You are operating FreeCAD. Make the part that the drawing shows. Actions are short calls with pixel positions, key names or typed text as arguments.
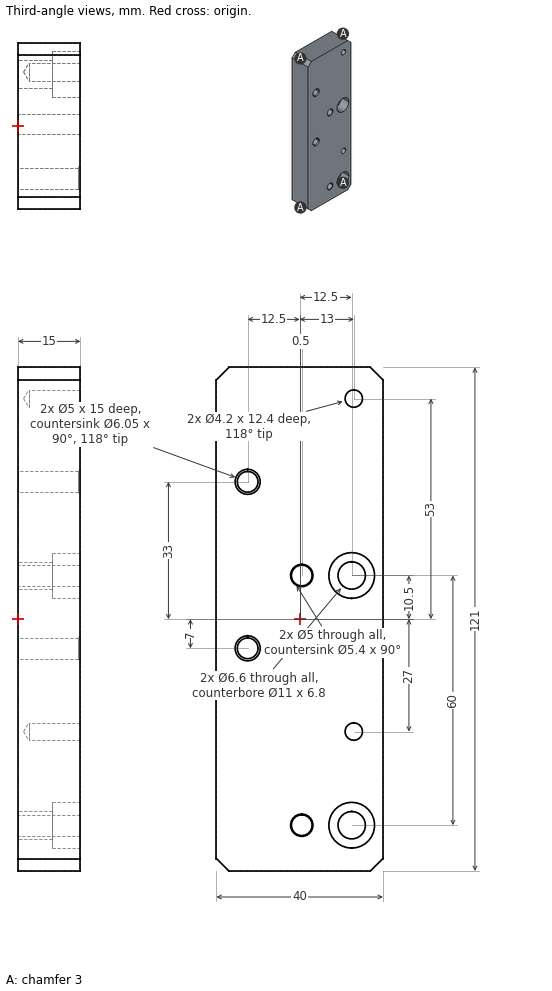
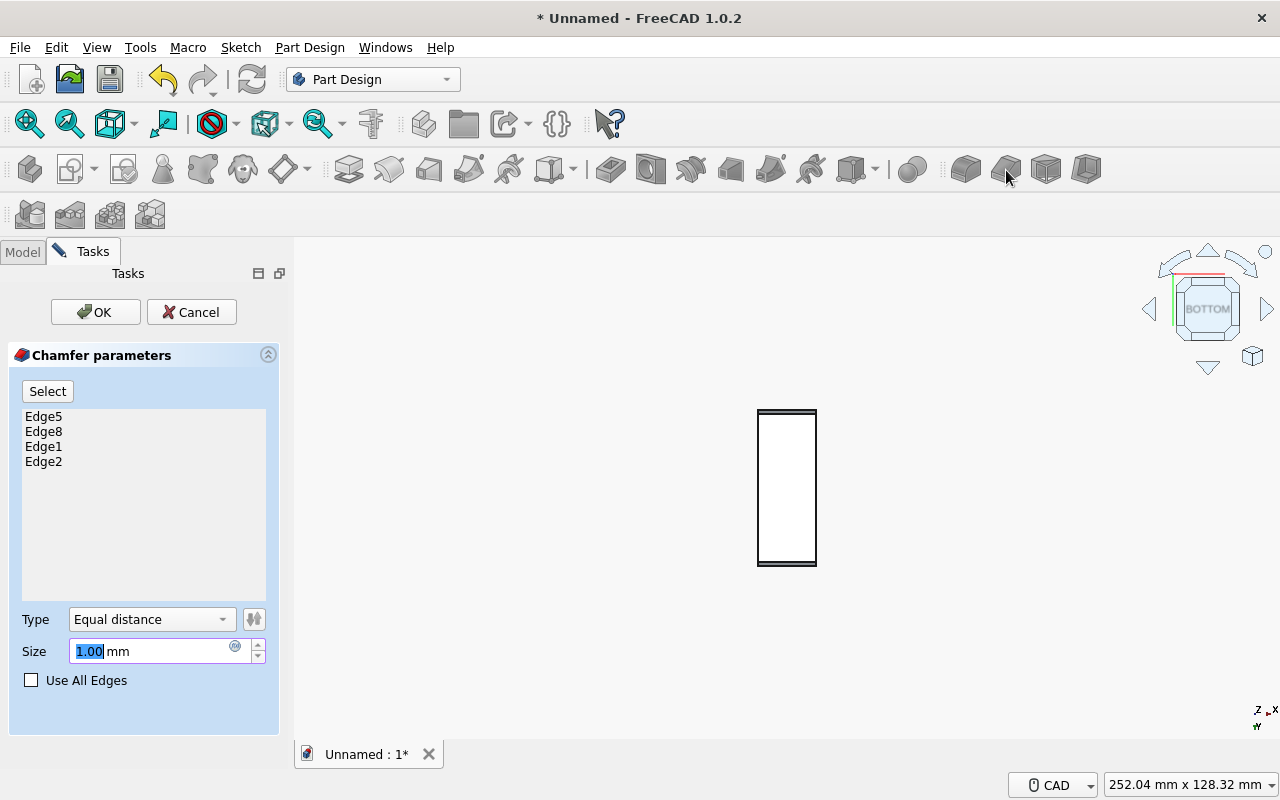
text(3)
key(Tab)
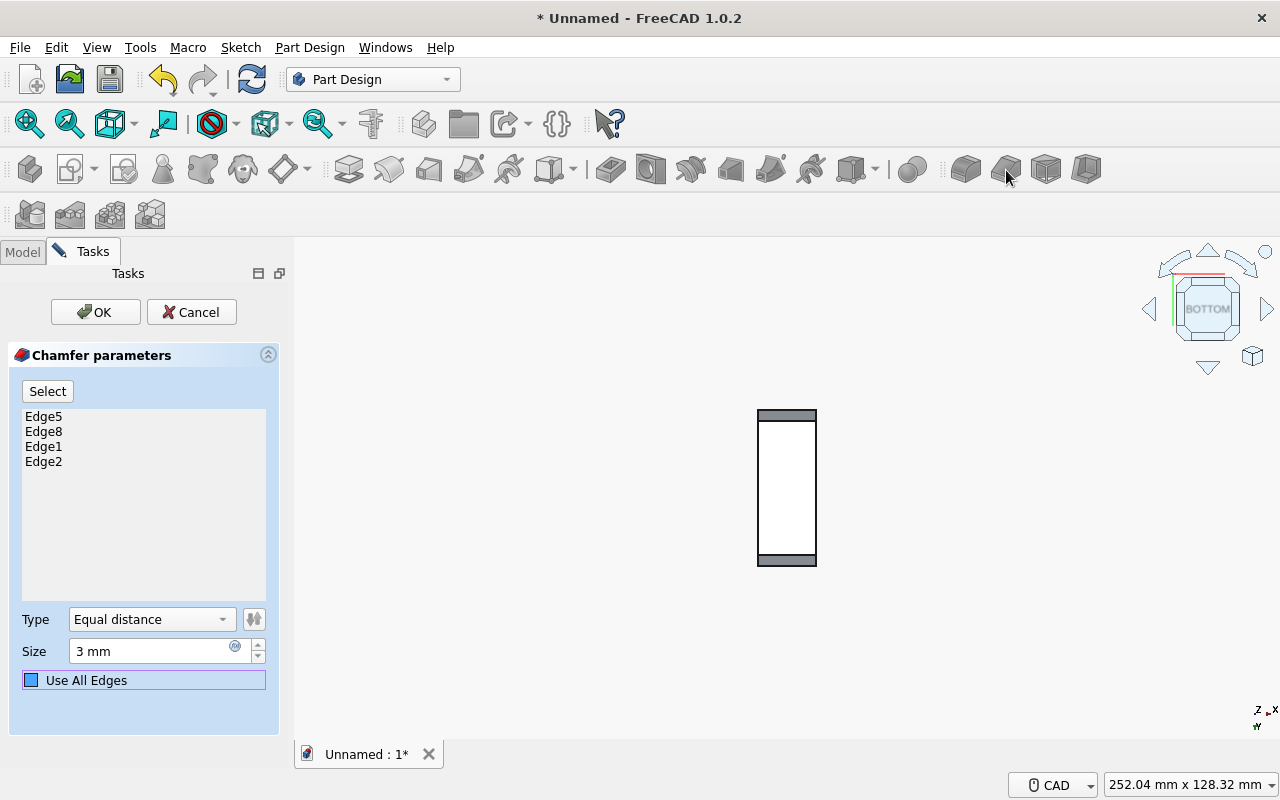
click(96, 312)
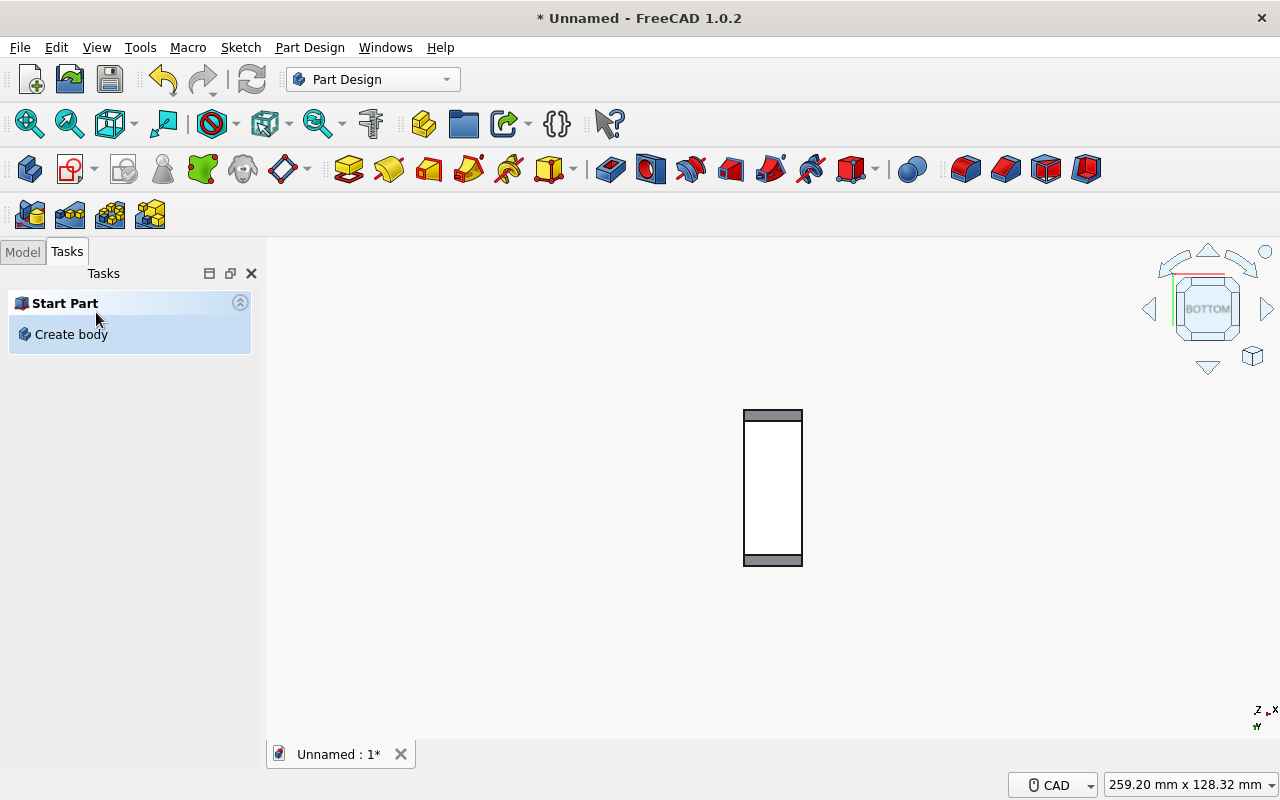
key(0)